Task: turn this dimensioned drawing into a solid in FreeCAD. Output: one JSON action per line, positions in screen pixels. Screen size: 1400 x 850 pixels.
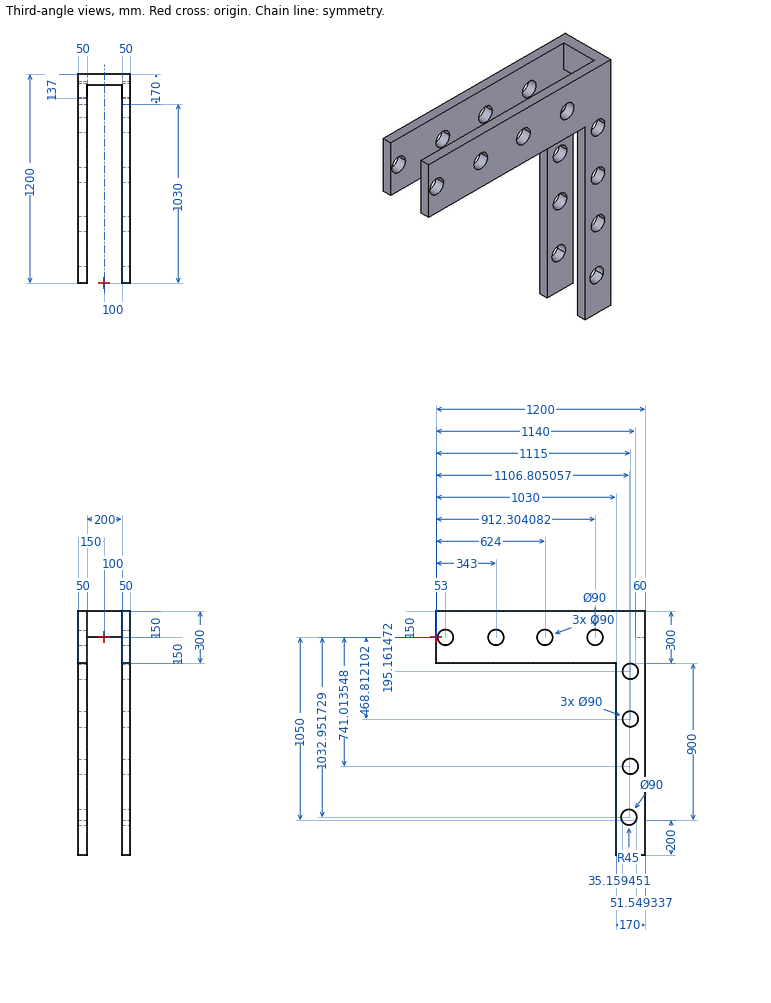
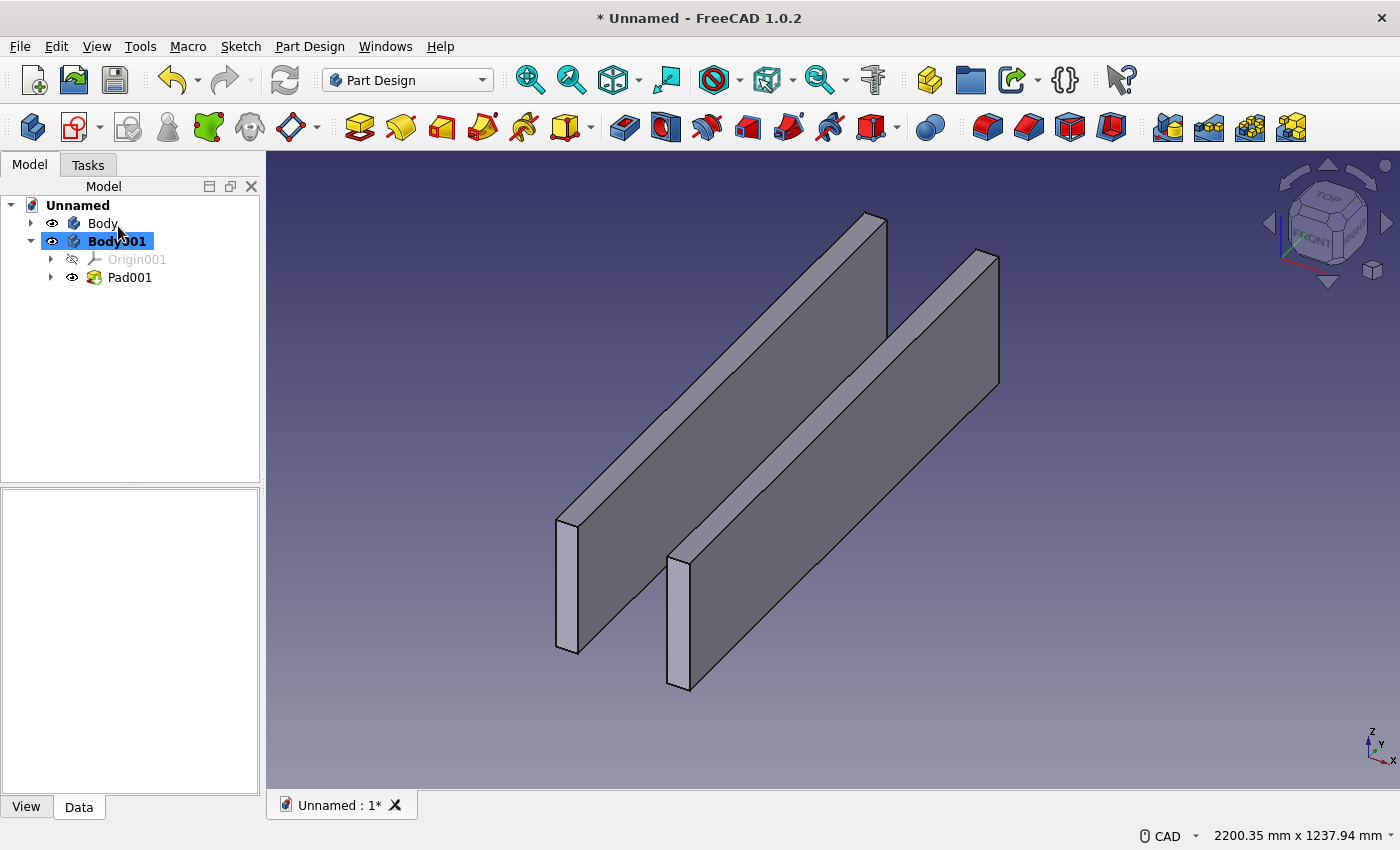
{"action": "double_click", "coordinate": [97, 223]}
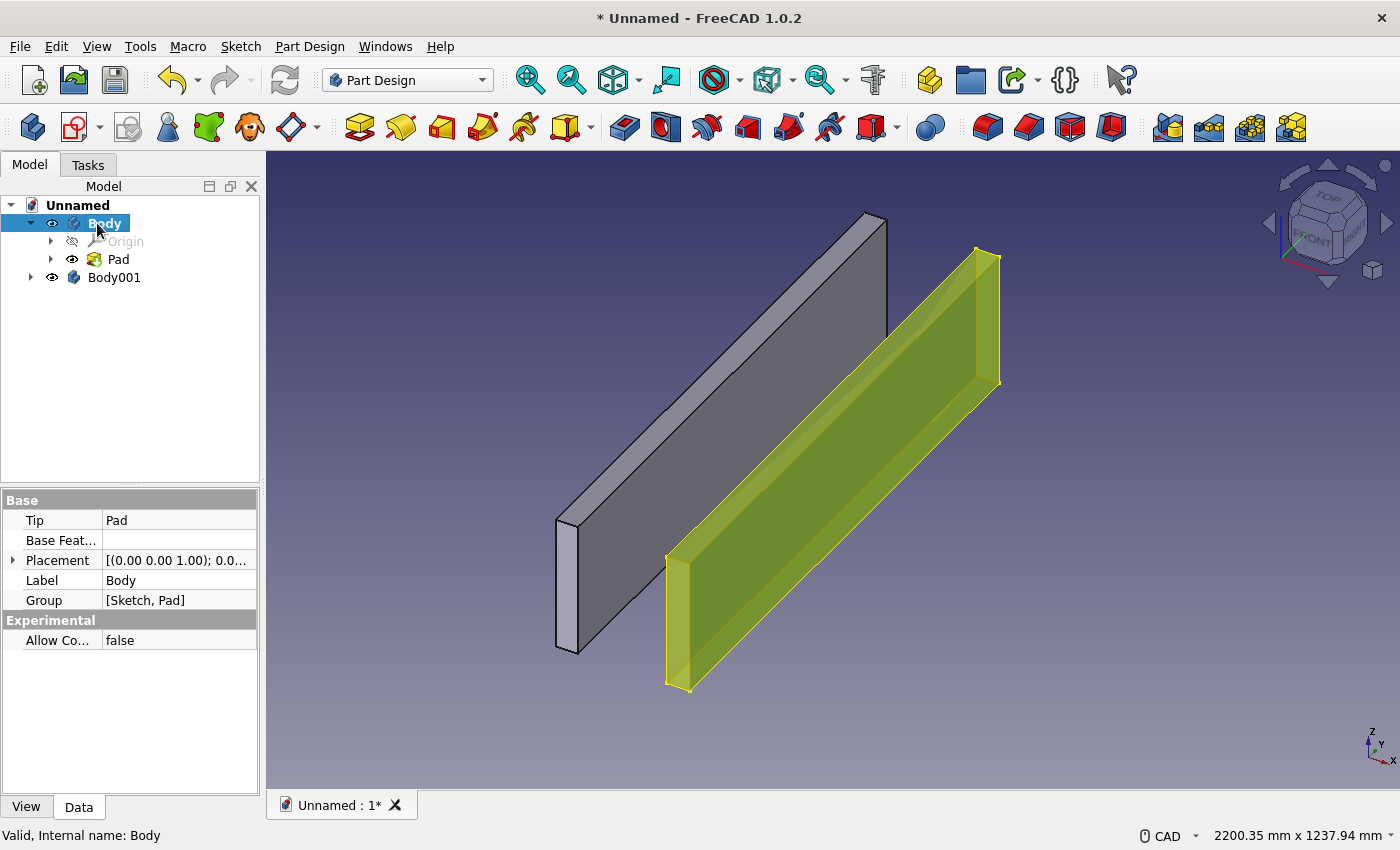
{"action": "left_click", "coordinate": [97, 223]}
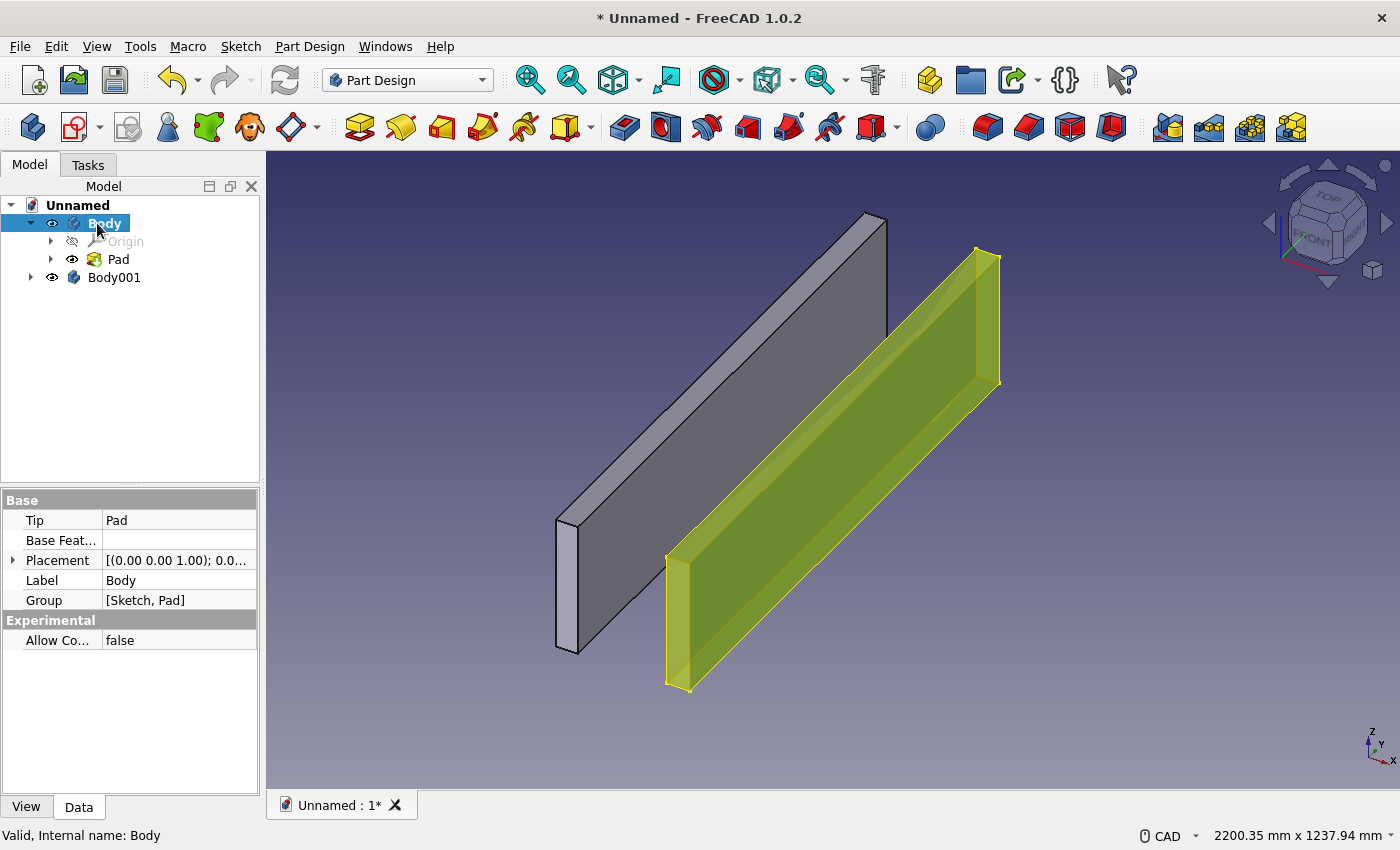
{"action": "left_click", "coordinate": [148, 640]}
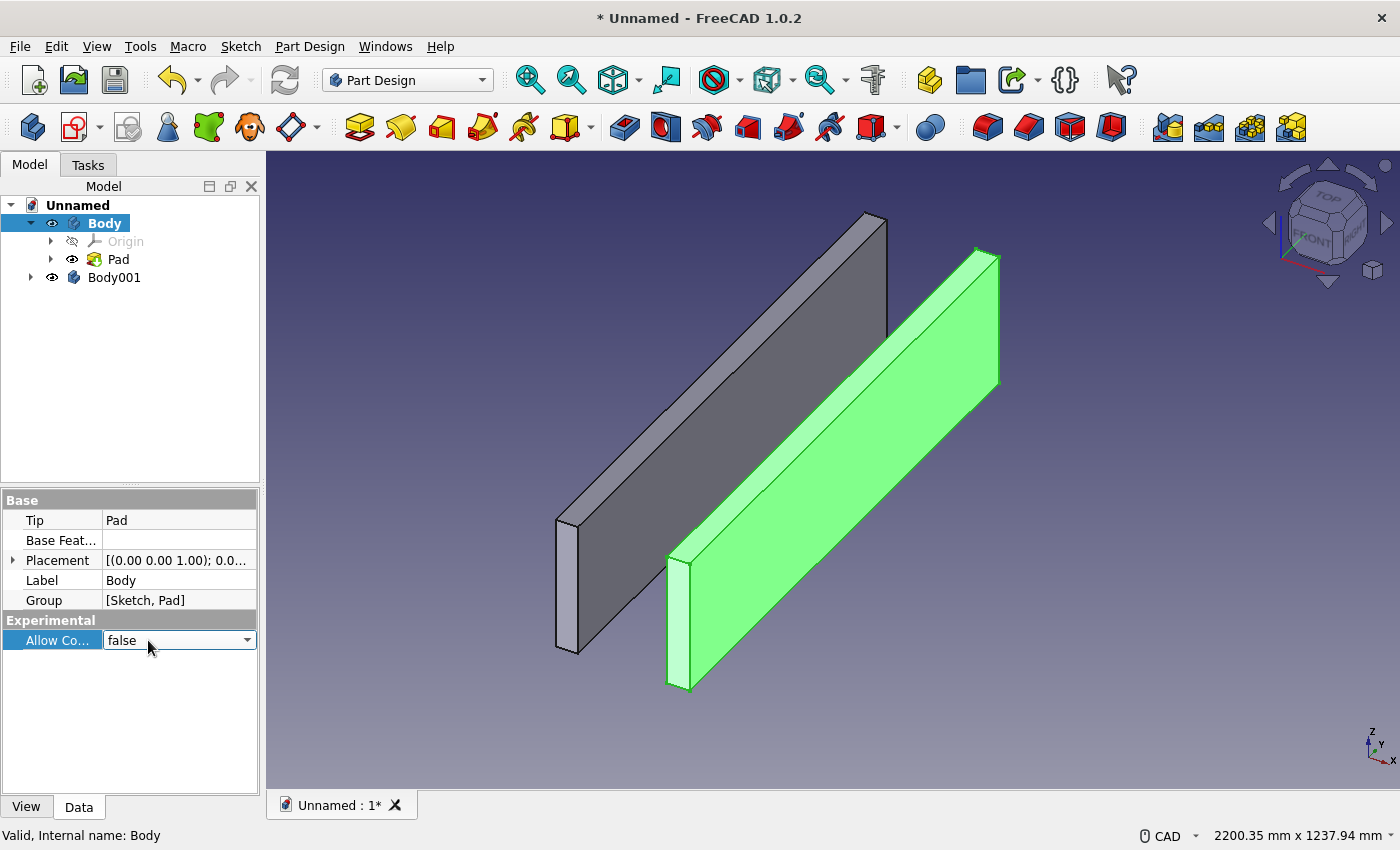
{"action": "left_click", "coordinate": [148, 640]}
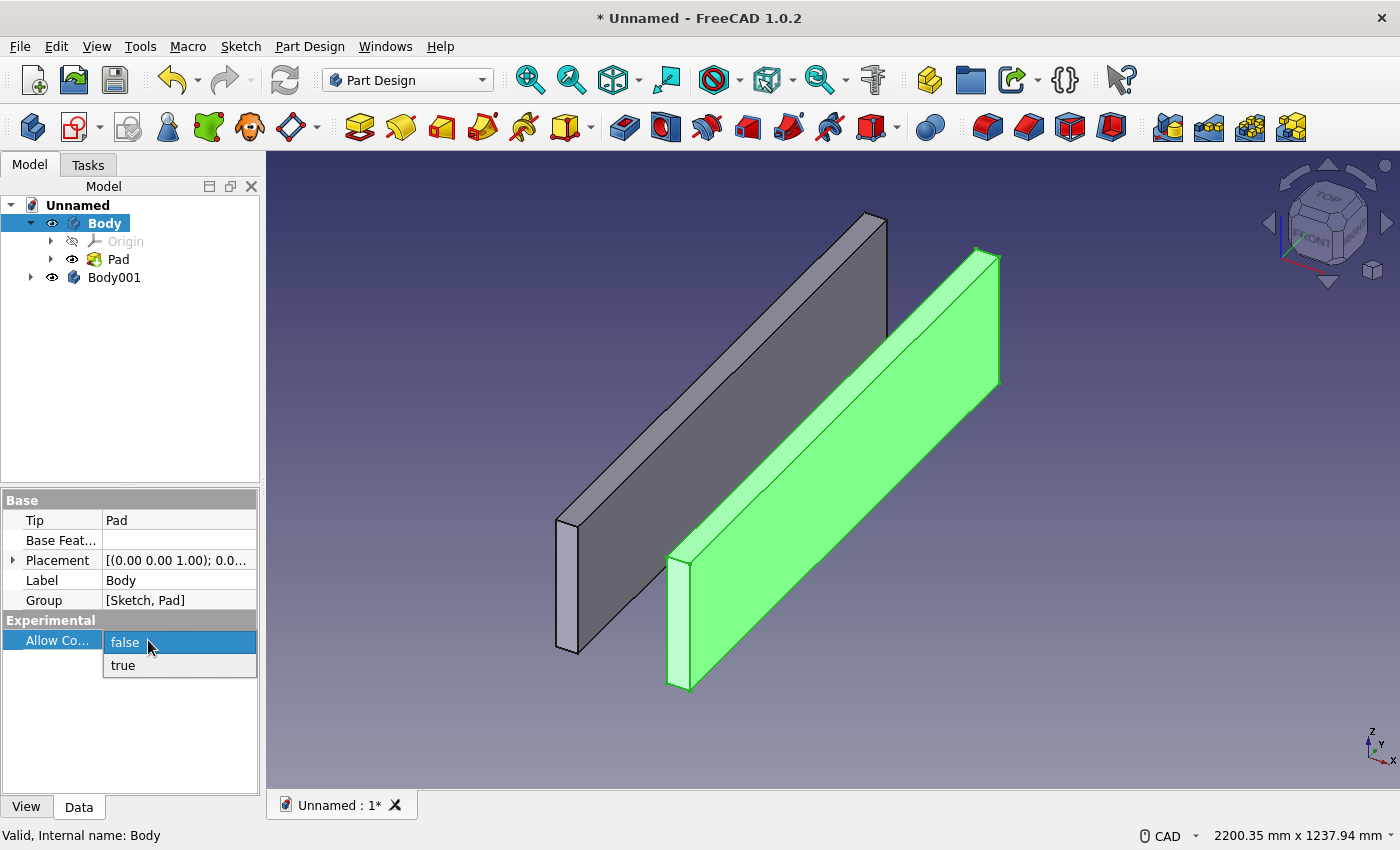
{"action": "left_click", "coordinate": [178, 666]}
{"action": "key", "text": "Return"}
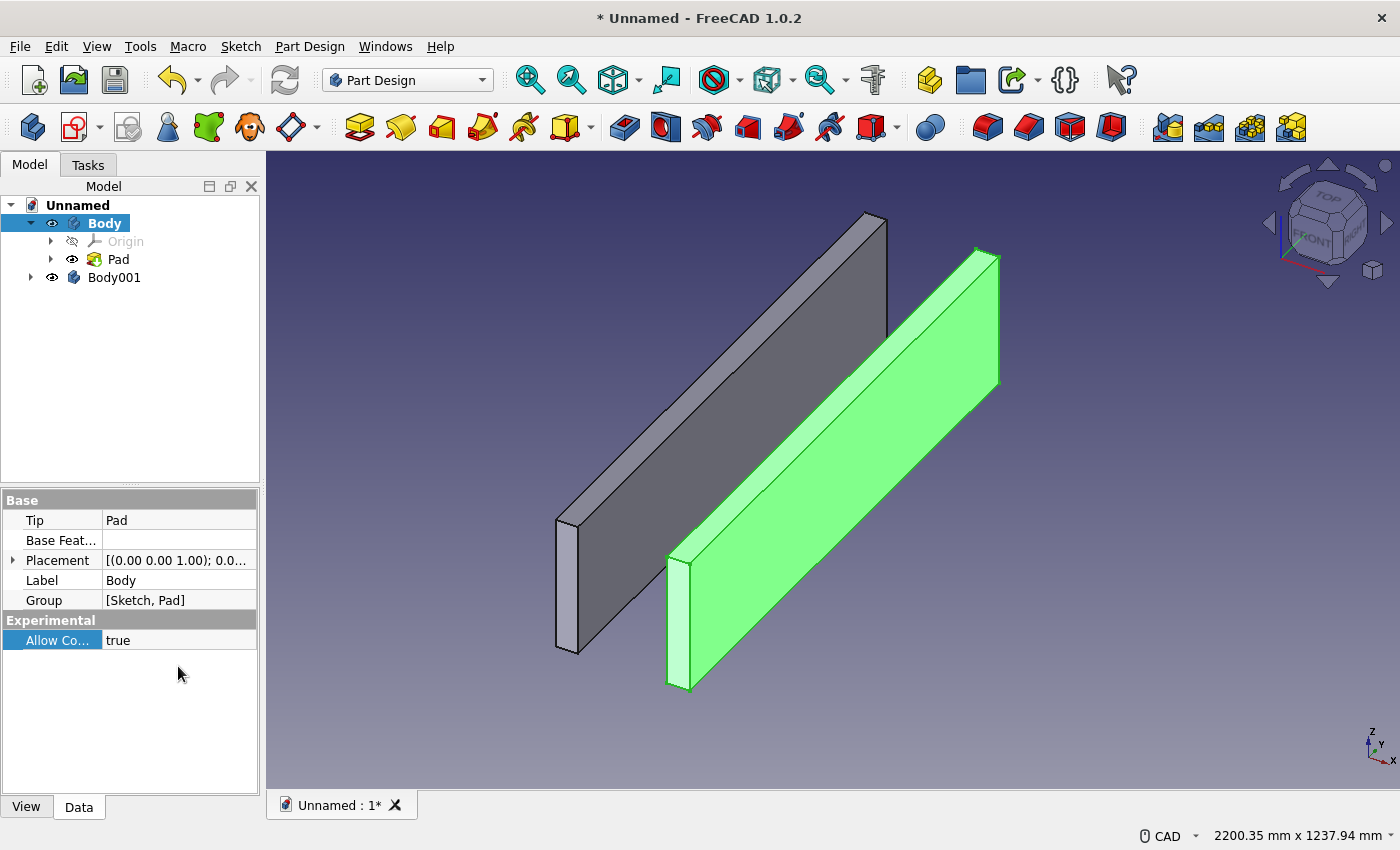
{"action": "left_click", "coordinate": [97, 277]}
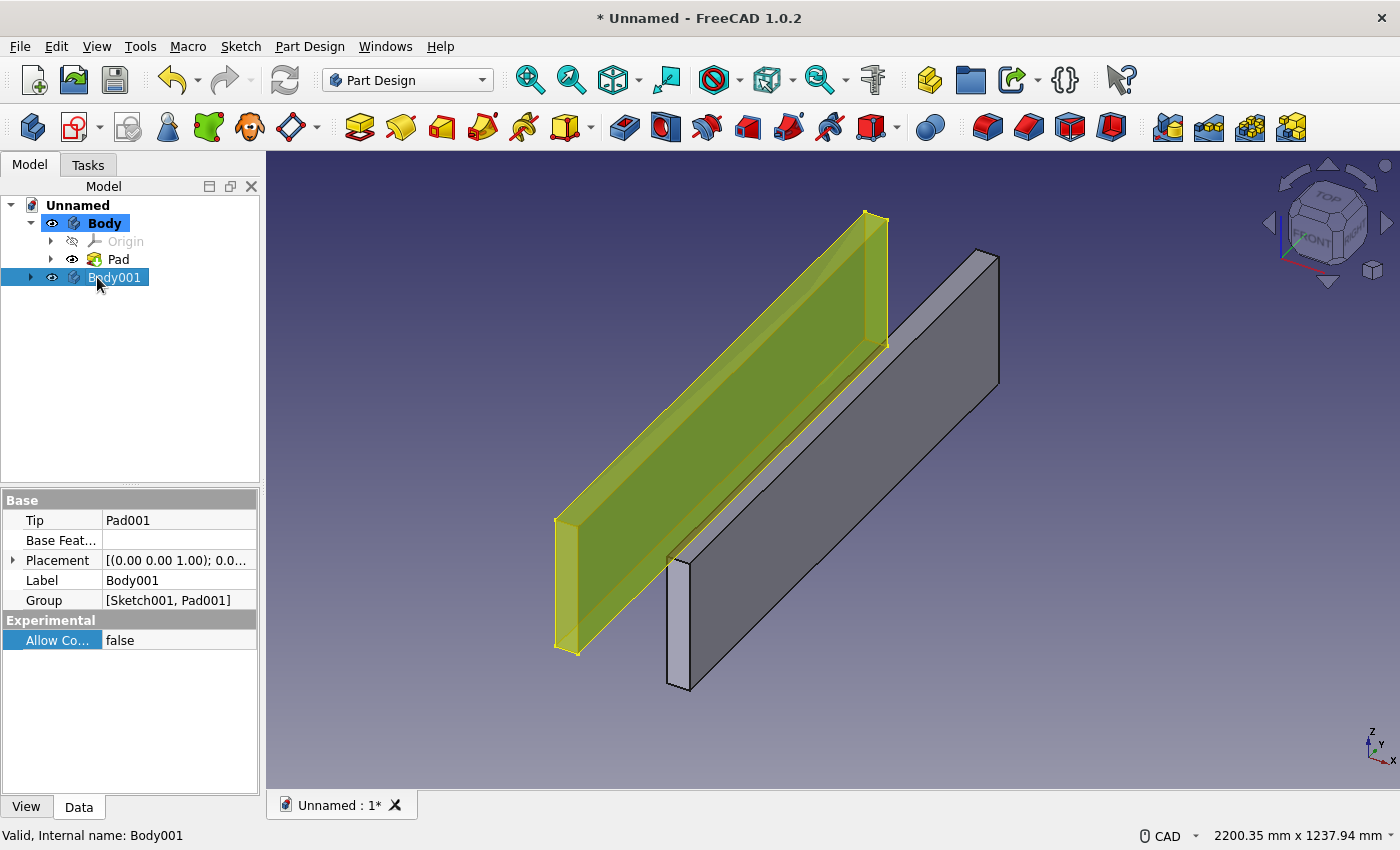
{"action": "left_click", "coordinate": [931, 128]}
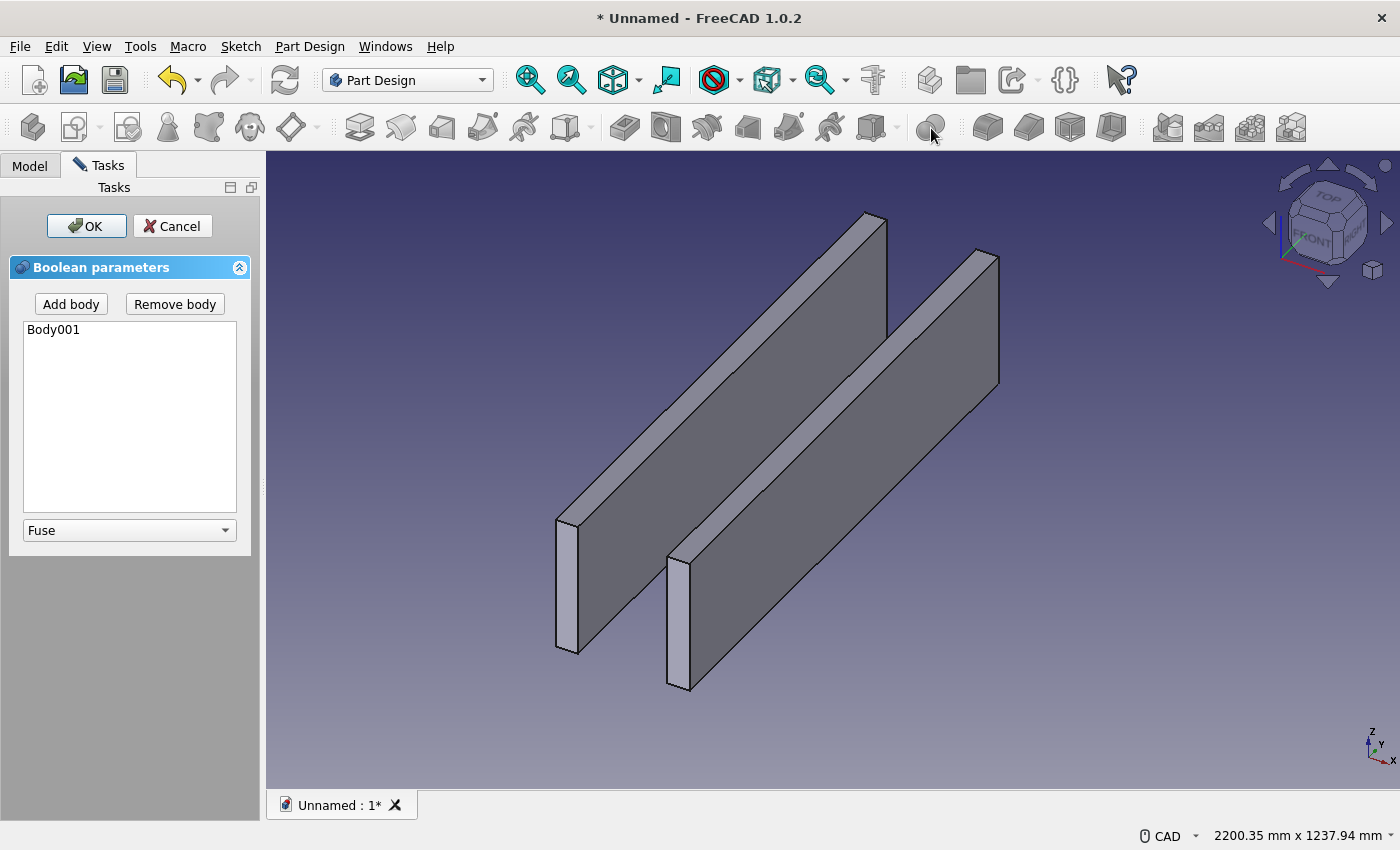
{"action": "left_click", "coordinate": [87, 226]}